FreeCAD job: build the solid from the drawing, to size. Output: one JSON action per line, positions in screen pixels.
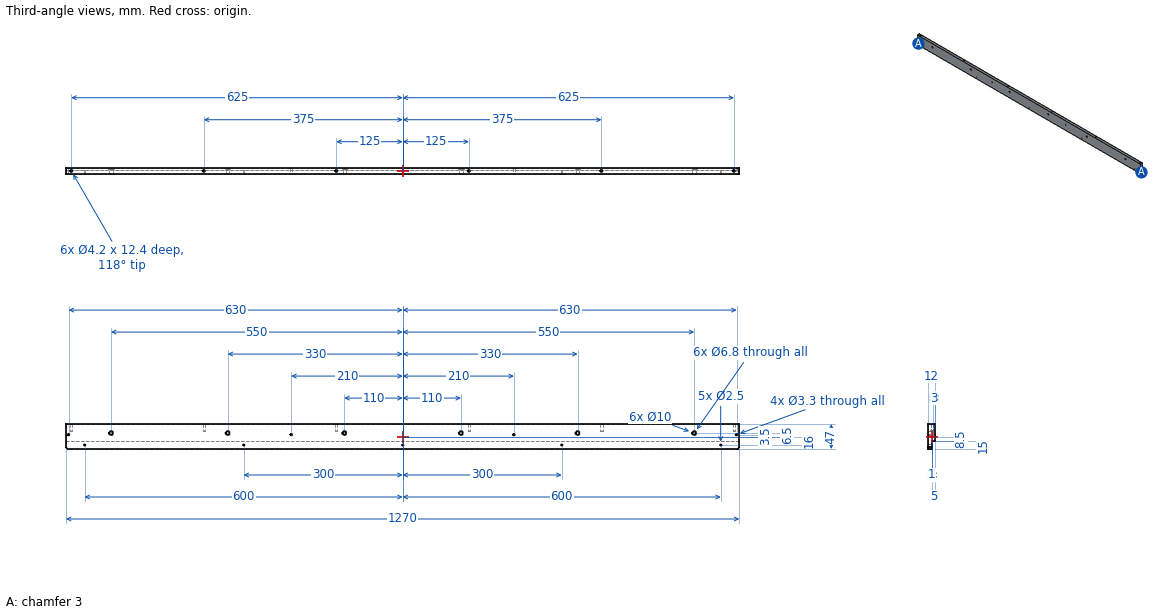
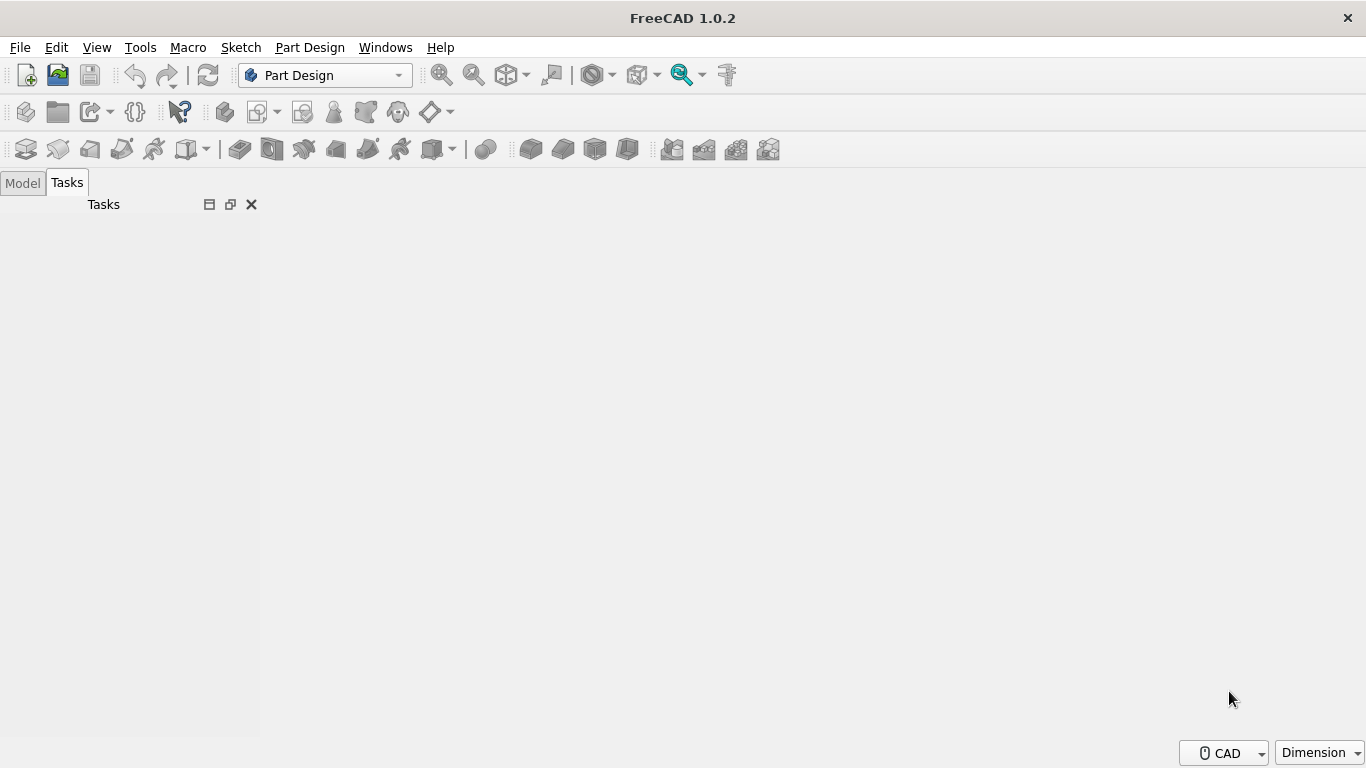
{"action": "left_click", "coordinate": [26, 76]}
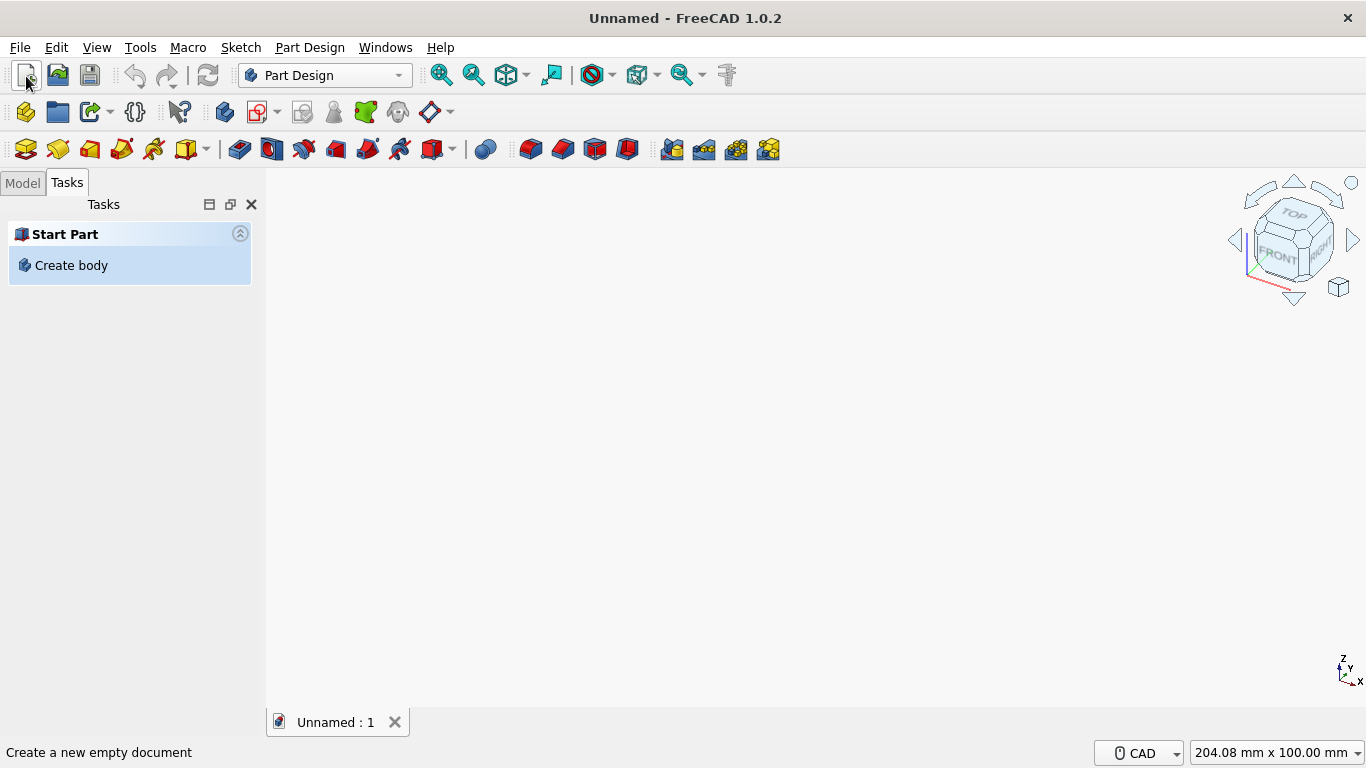
{"action": "left_click", "coordinate": [258, 112]}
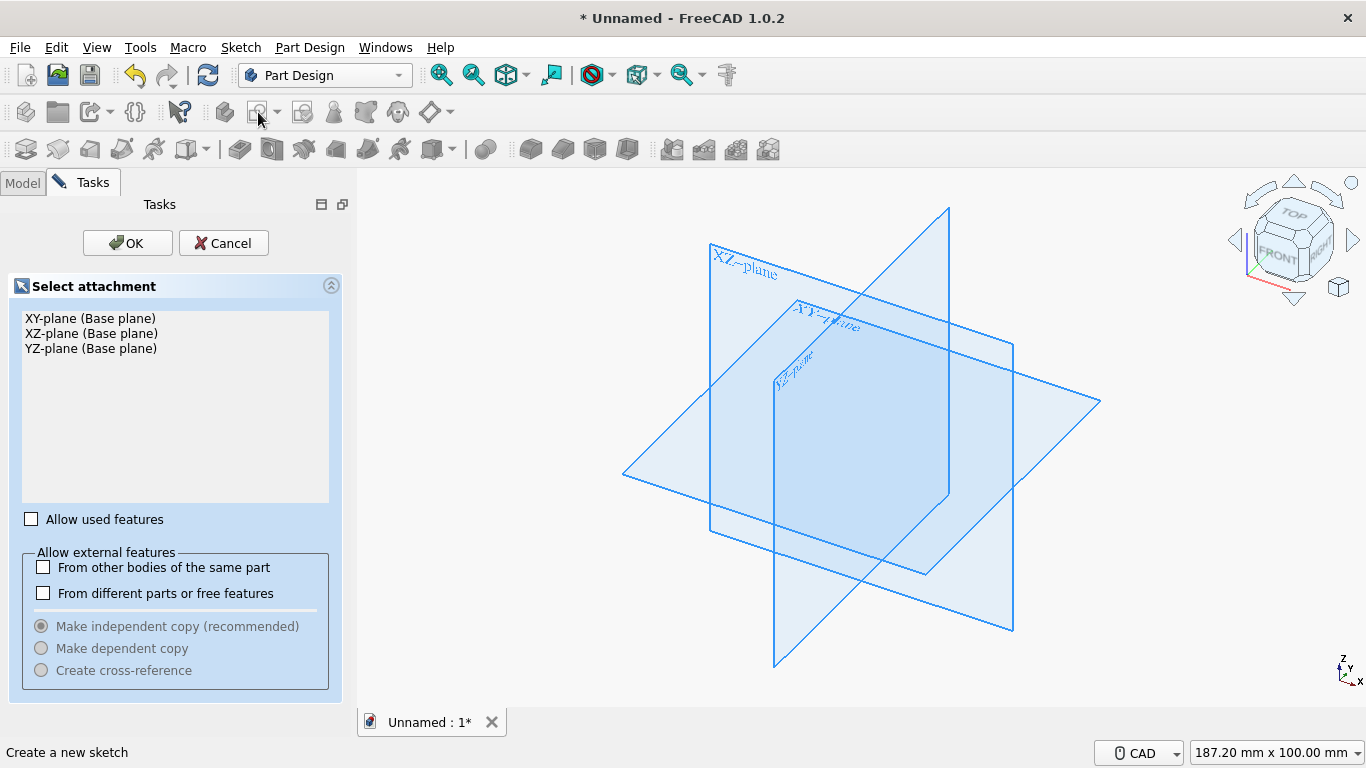
{"action": "left_click", "coordinate": [82, 334]}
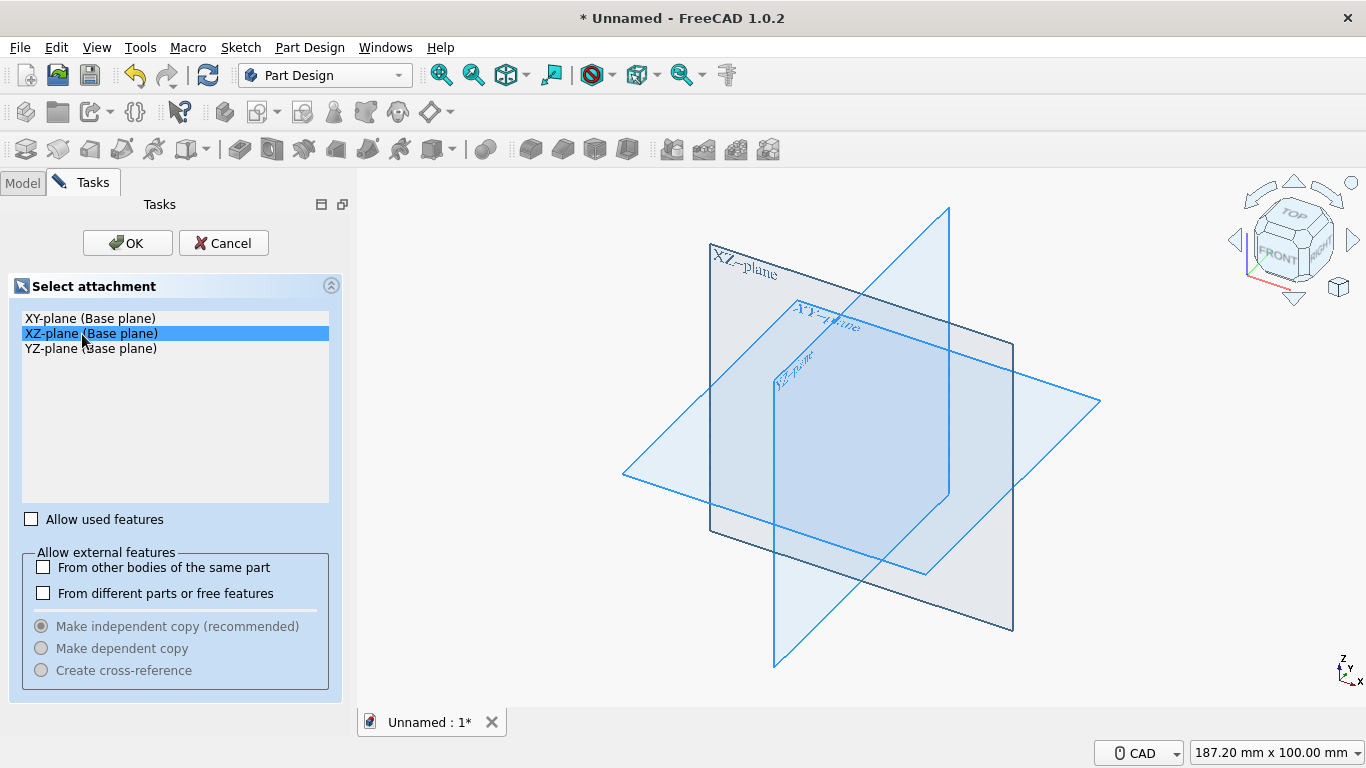
{"action": "left_click", "coordinate": [128, 243]}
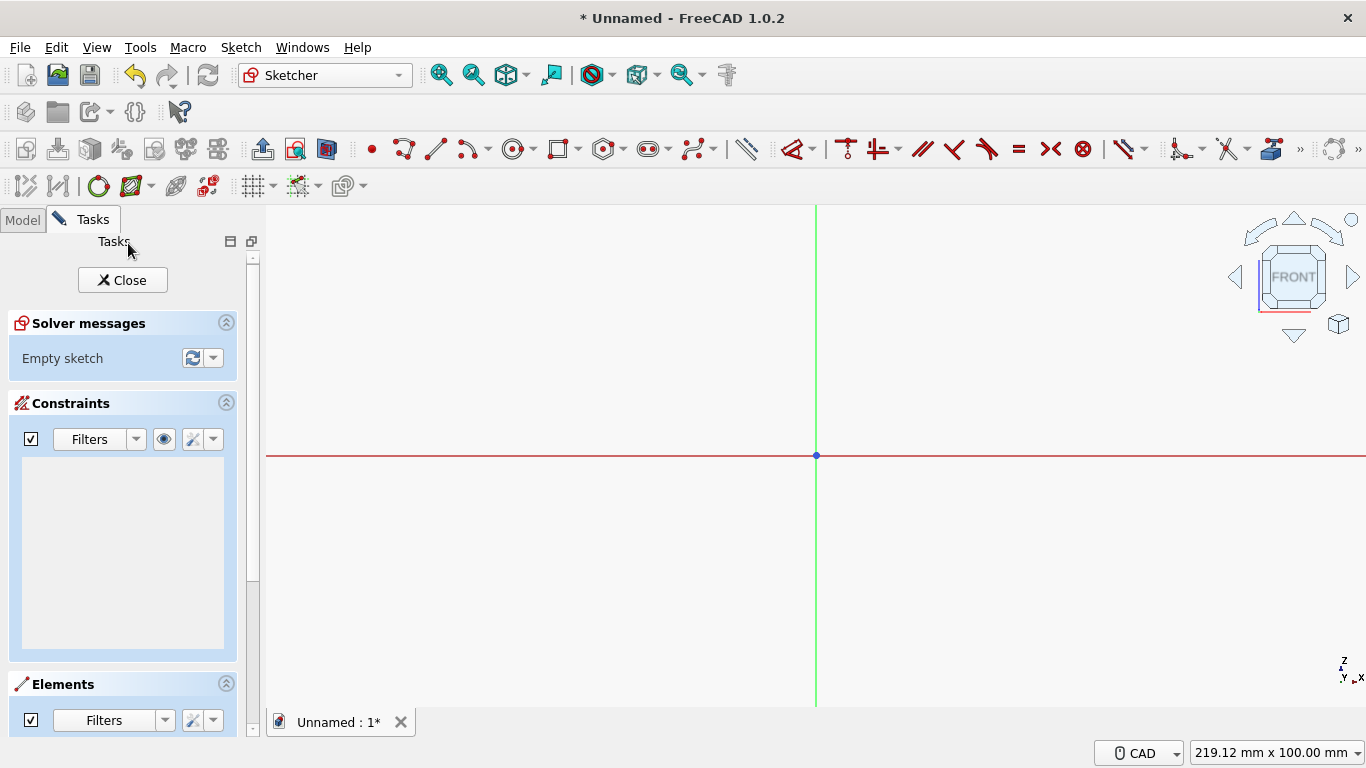
{"action": "scroll", "coordinate": [739, 456], "scroll_direction": "down", "scroll_amount": 11}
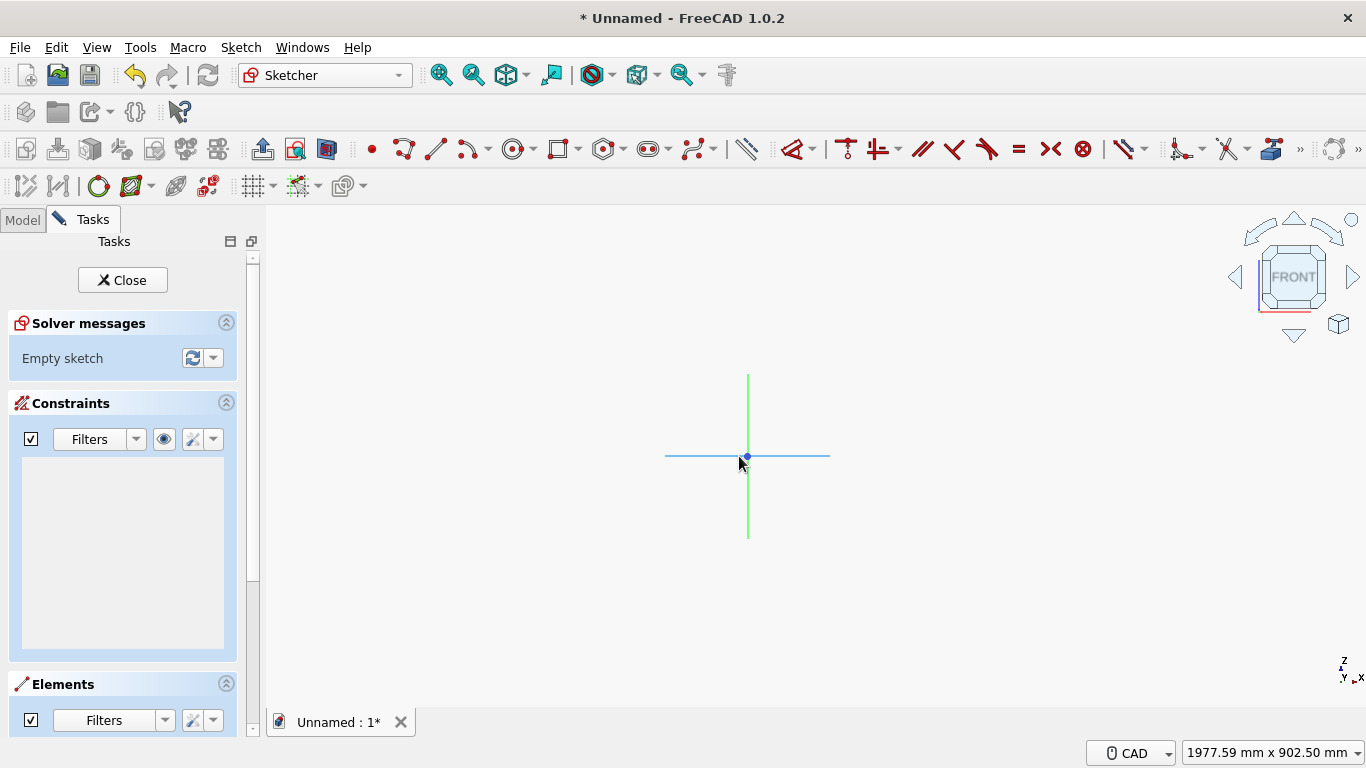
{"action": "left_click", "coordinate": [580, 150]}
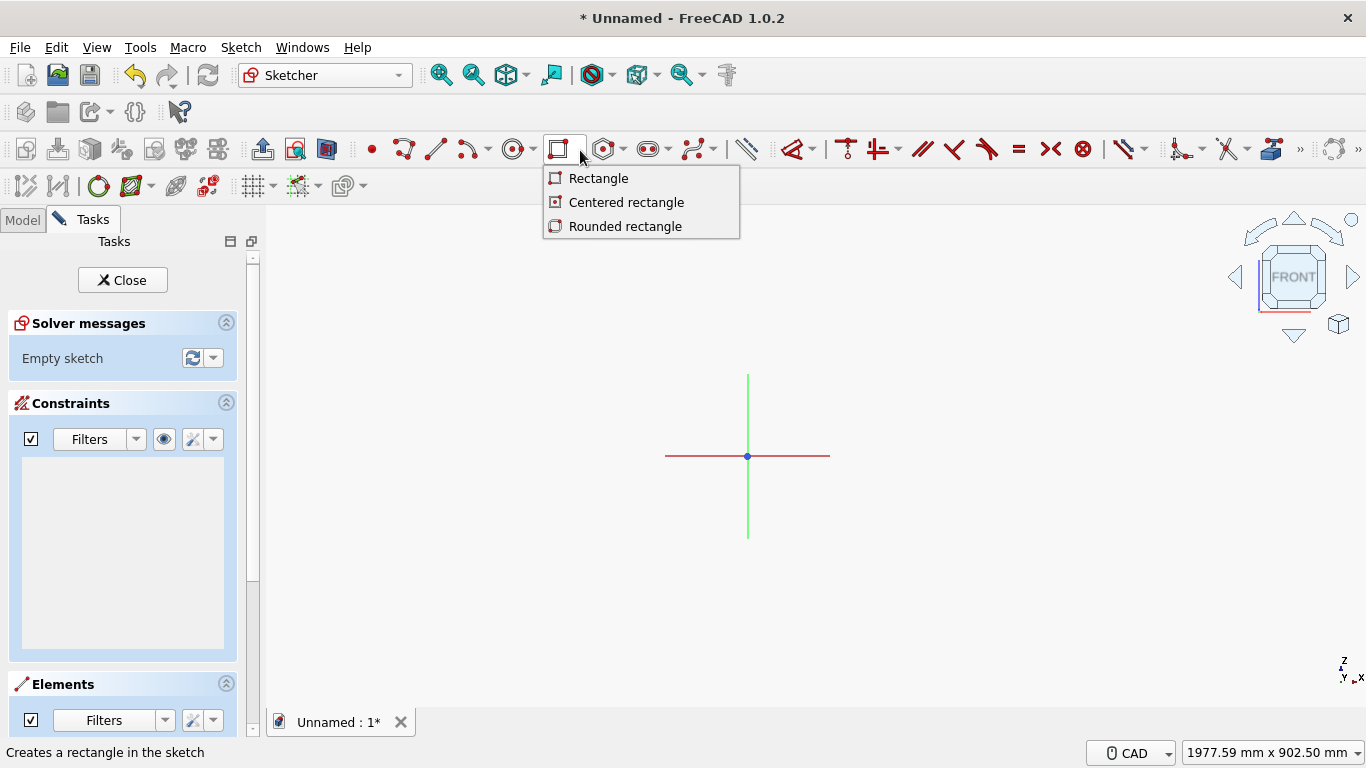
{"action": "left_click", "coordinate": [642, 202]}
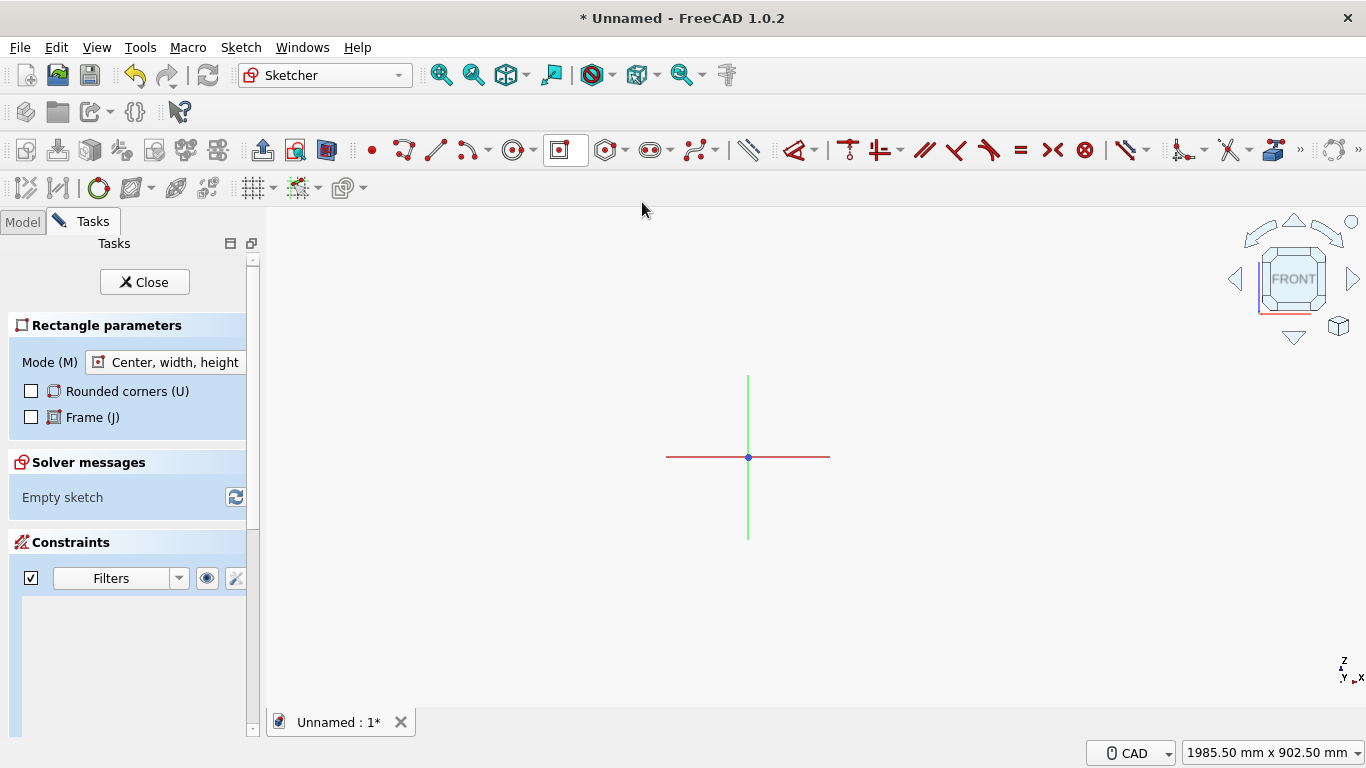
{"action": "left_click", "coordinate": [748, 457]}
{"action": "mouse_move", "coordinate": [1100, 444]}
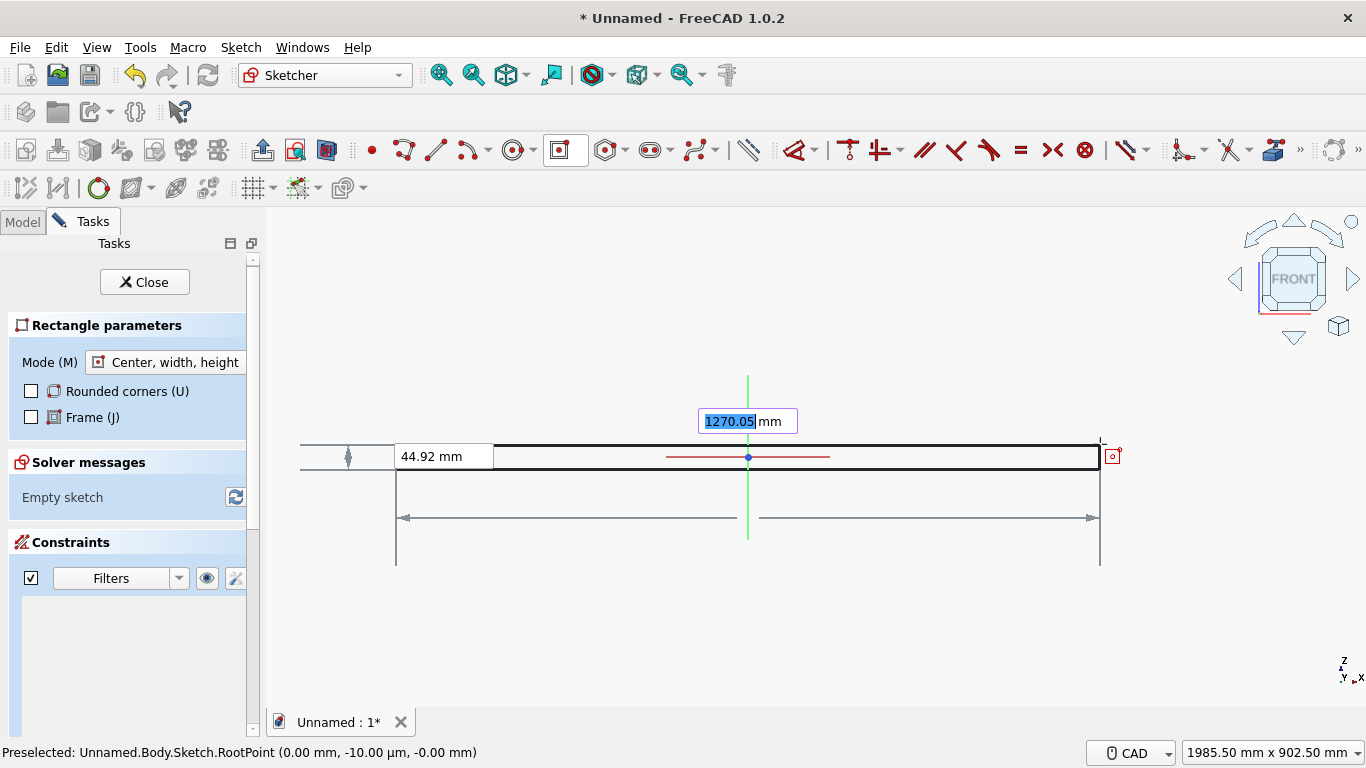
{"action": "type", "text": "1270"}
{"action": "key", "text": "Tab"}
{"action": "type", "text": "47"}
{"action": "key", "text": "Return"}
{"action": "key", "text": "Escape"}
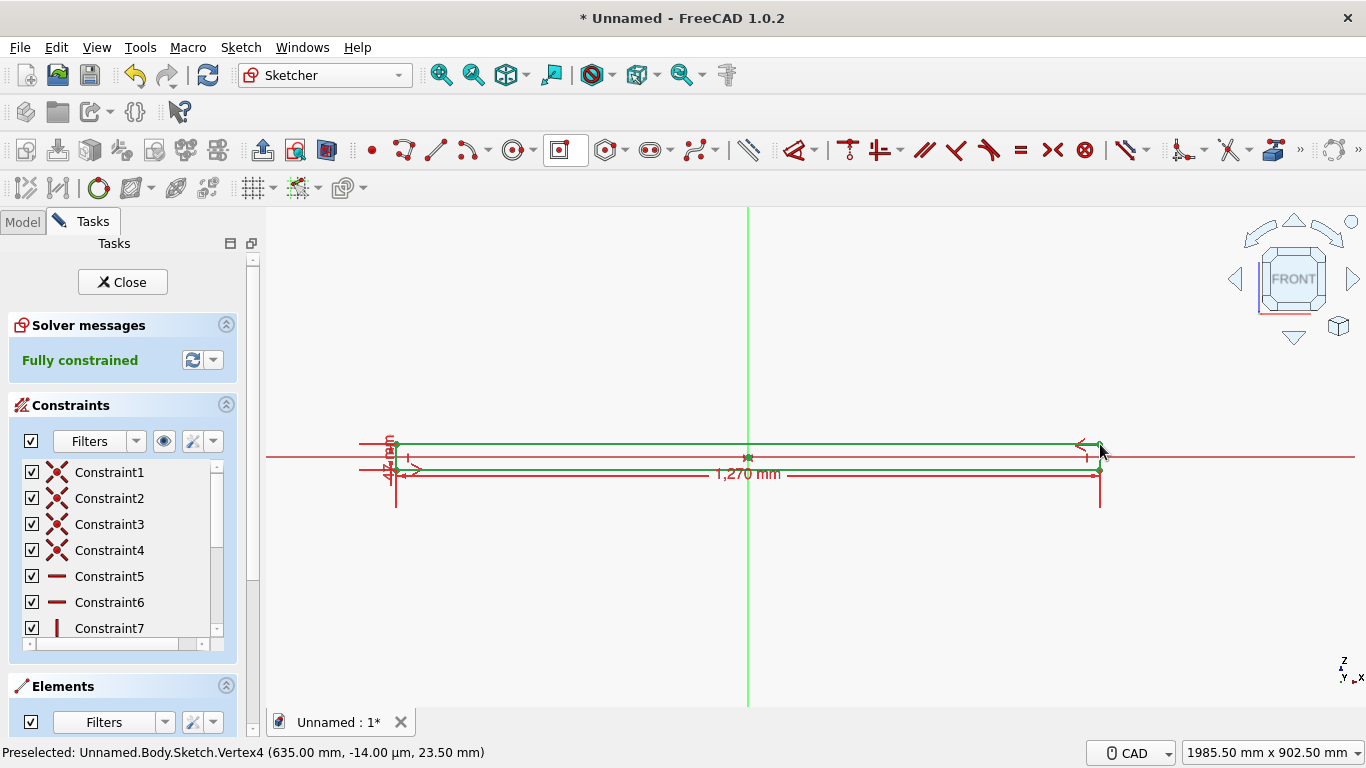
{"action": "left_click", "coordinate": [123, 282]}